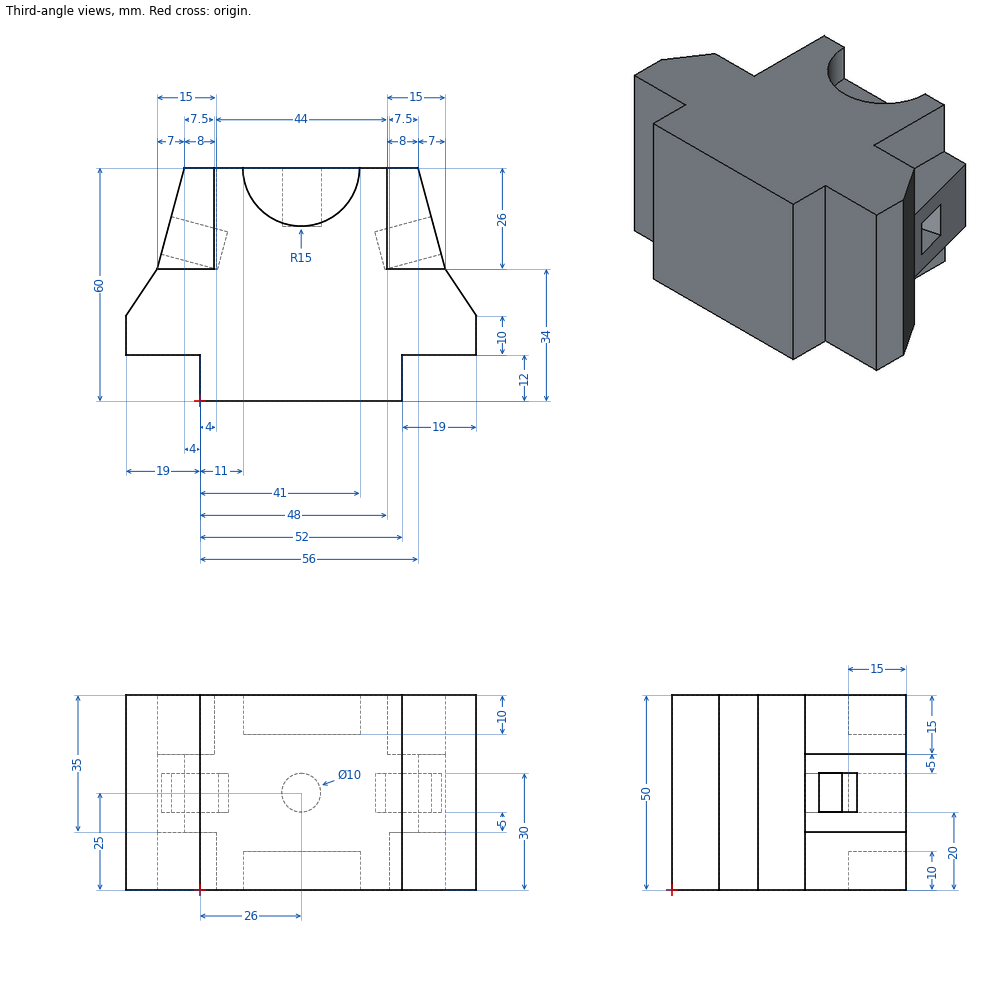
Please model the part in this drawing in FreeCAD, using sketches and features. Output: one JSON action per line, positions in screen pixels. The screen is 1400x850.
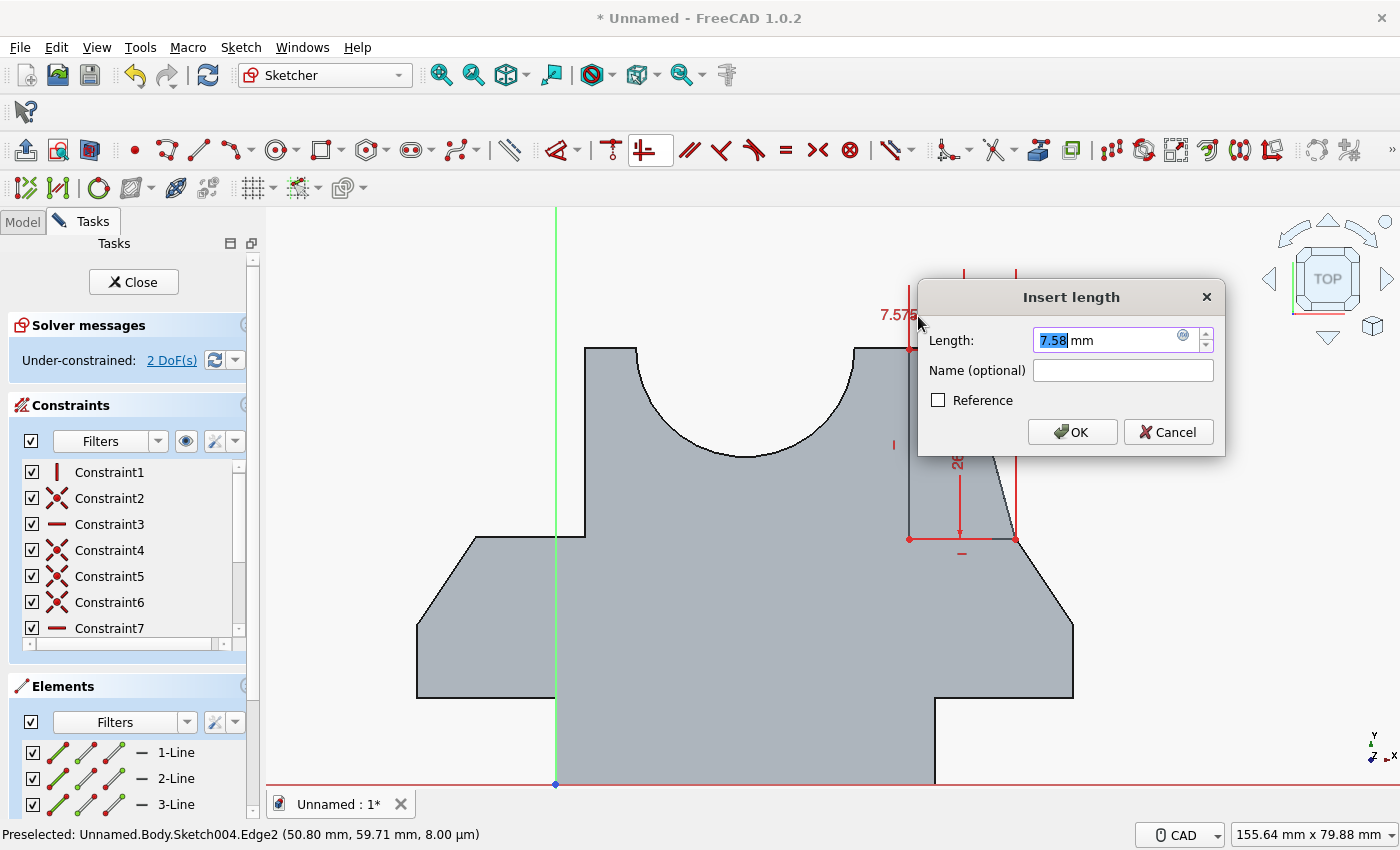
{"action": "type", "text": "7.5"}
{"action": "key", "text": "Return"}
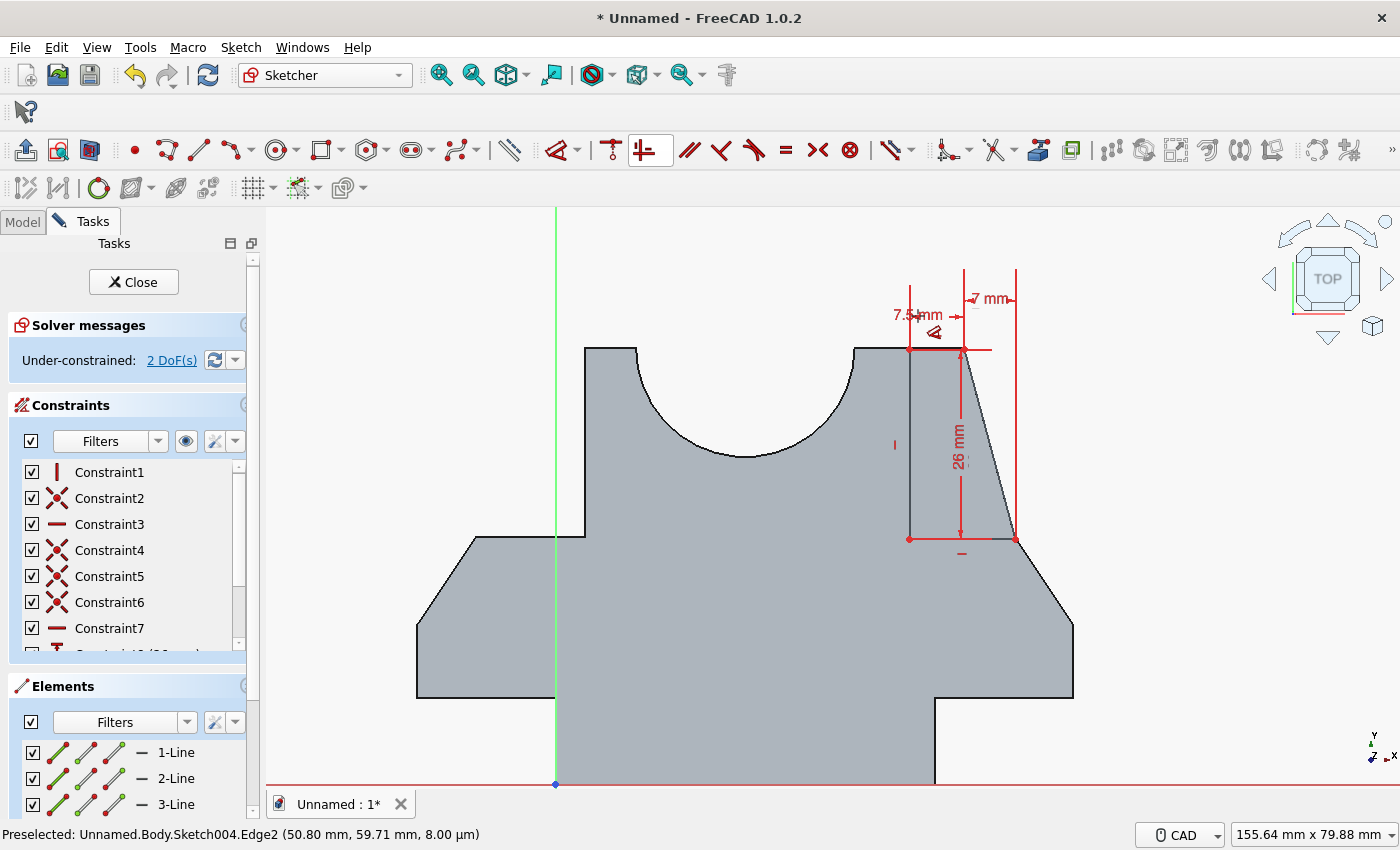
{"action": "left_click", "coordinate": [910, 539]}
{"action": "left_click", "coordinate": [522, 650]}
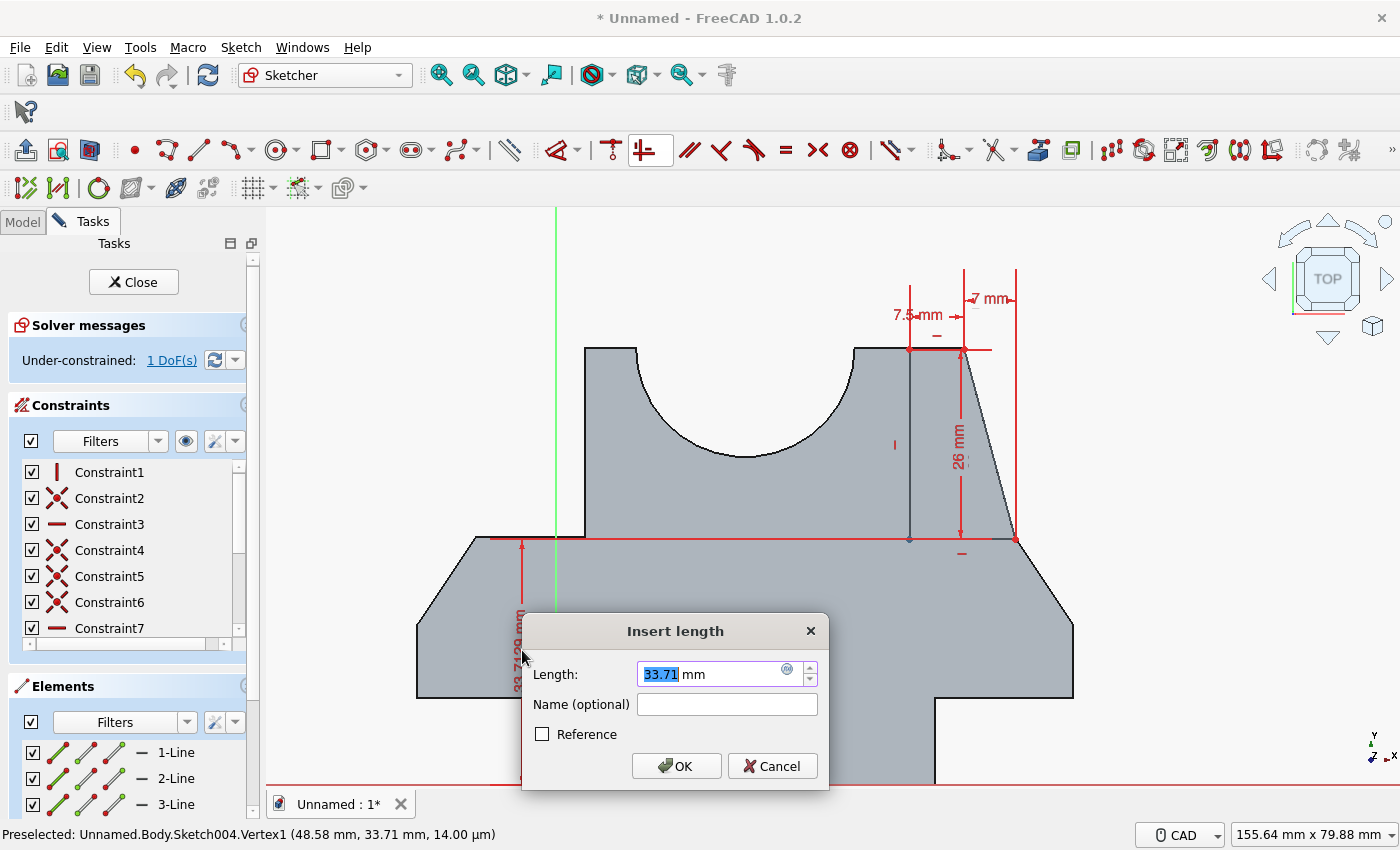
{"action": "type", "text": "34"}
{"action": "key", "text": "Return"}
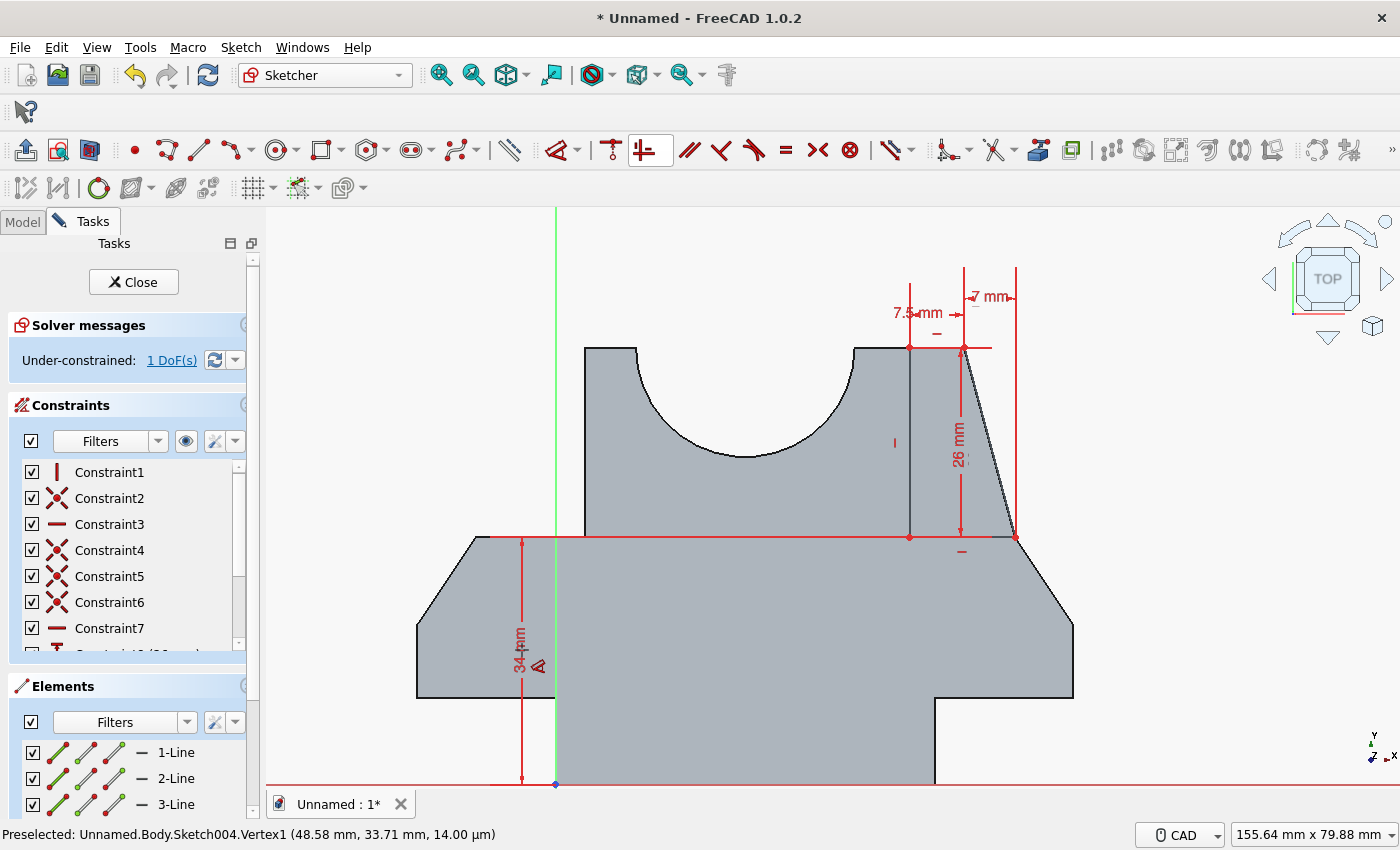
{"action": "left_click", "coordinate": [965, 348]}
{"action": "left_click", "coordinate": [760, 314]}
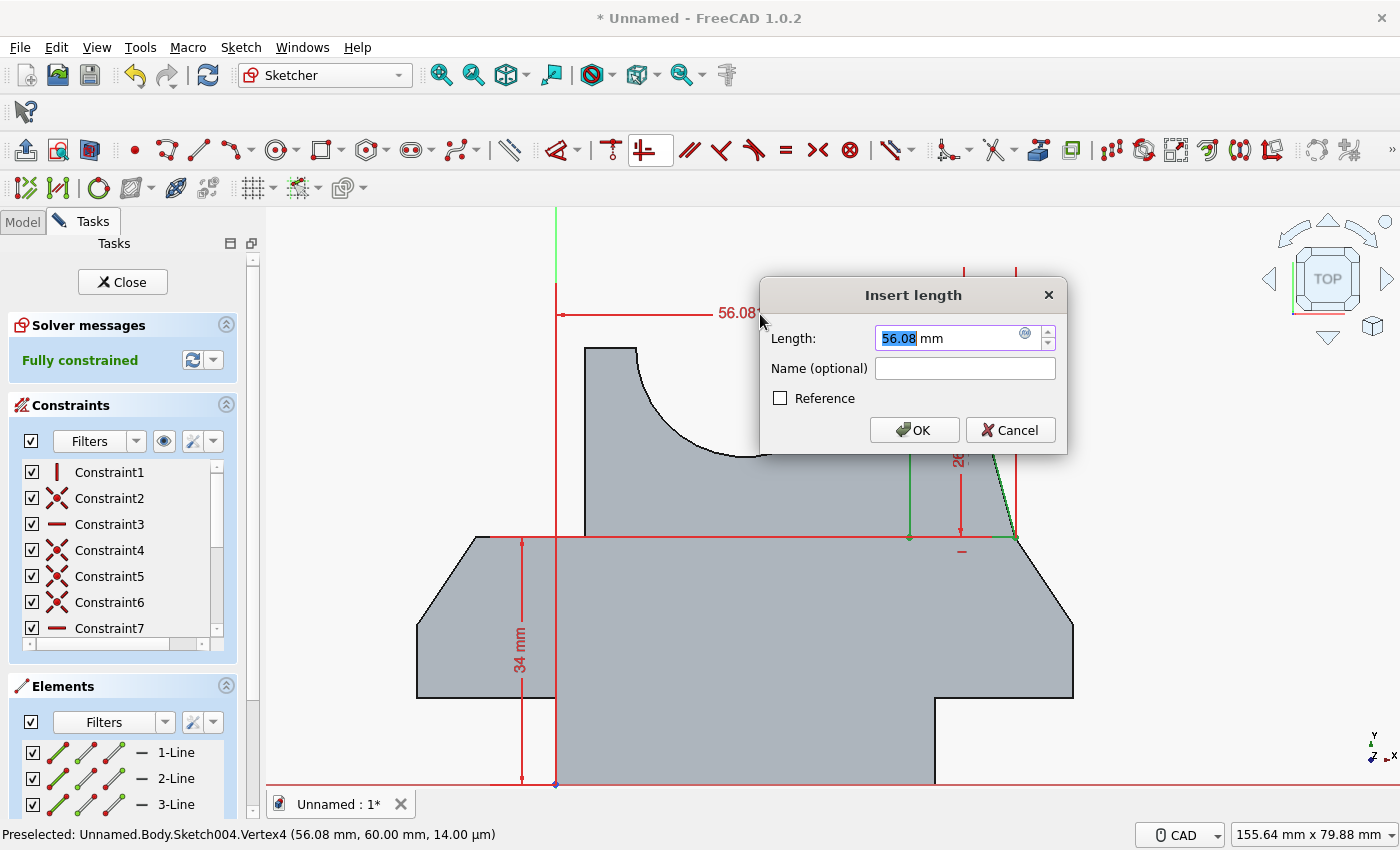
{"action": "type", "text": "56"}
{"action": "key", "text": "Return"}
{"action": "key", "text": "Escape"}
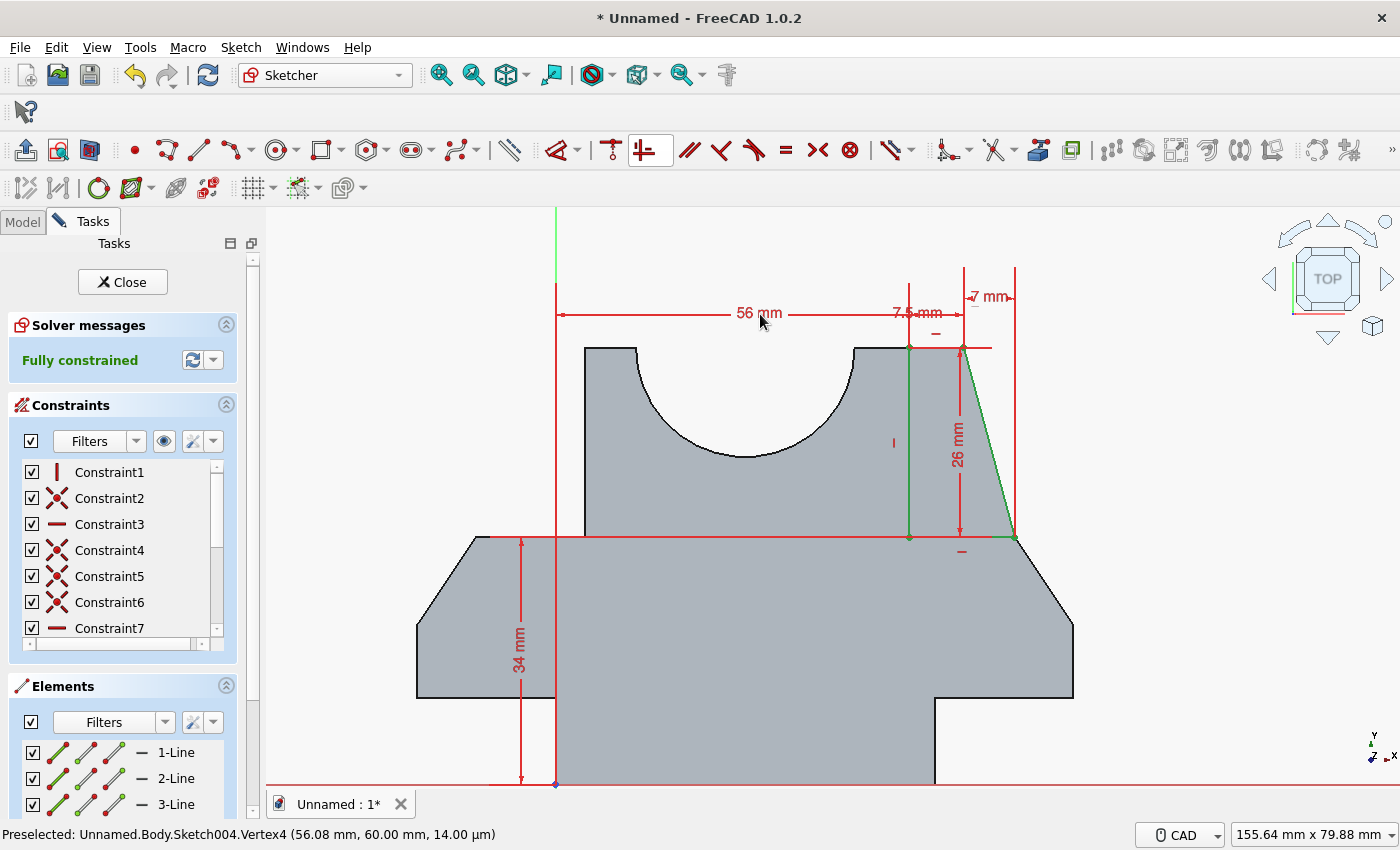
{"action": "left_click", "coordinate": [123, 282]}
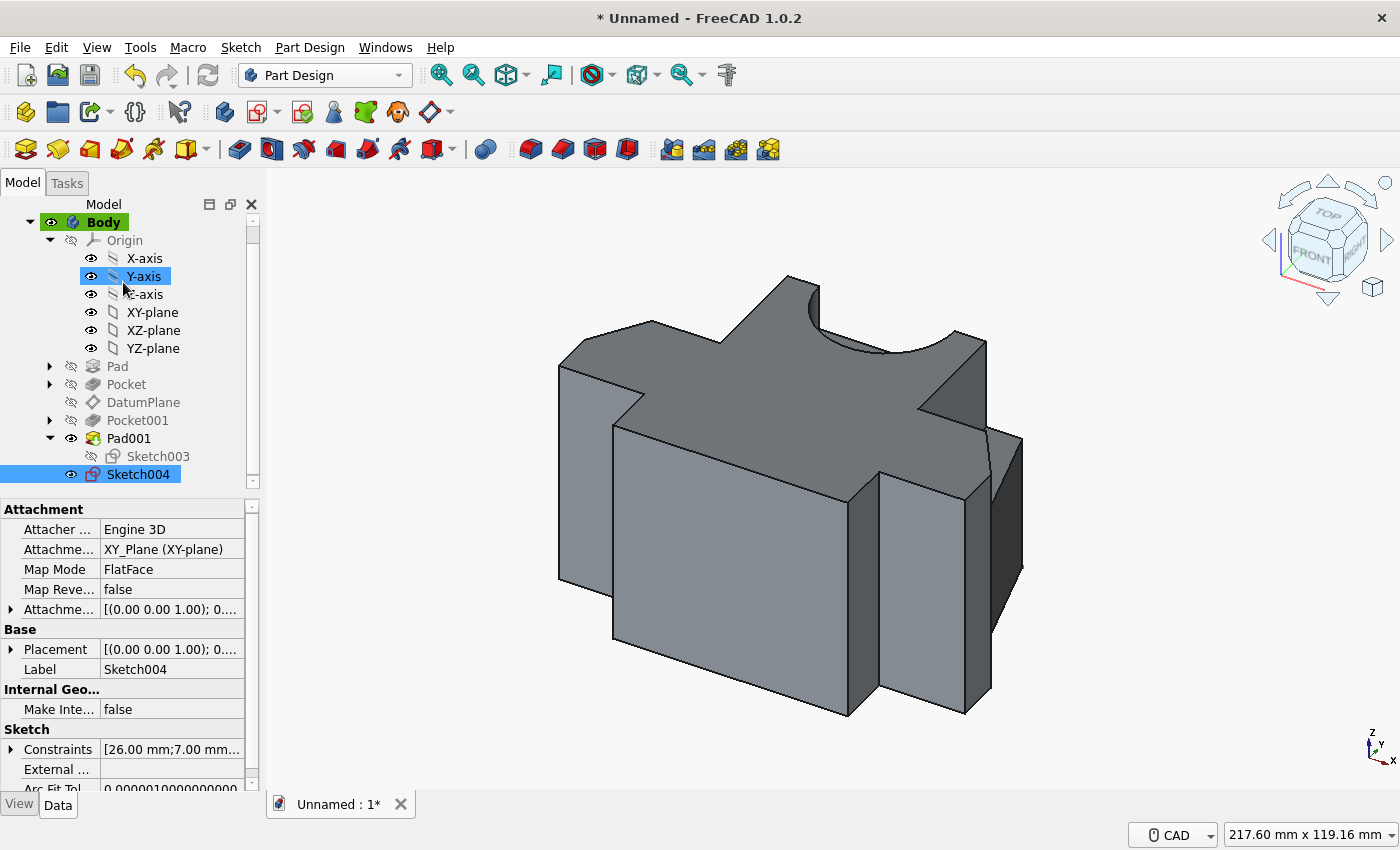
{"action": "left_click", "coordinate": [240, 150]}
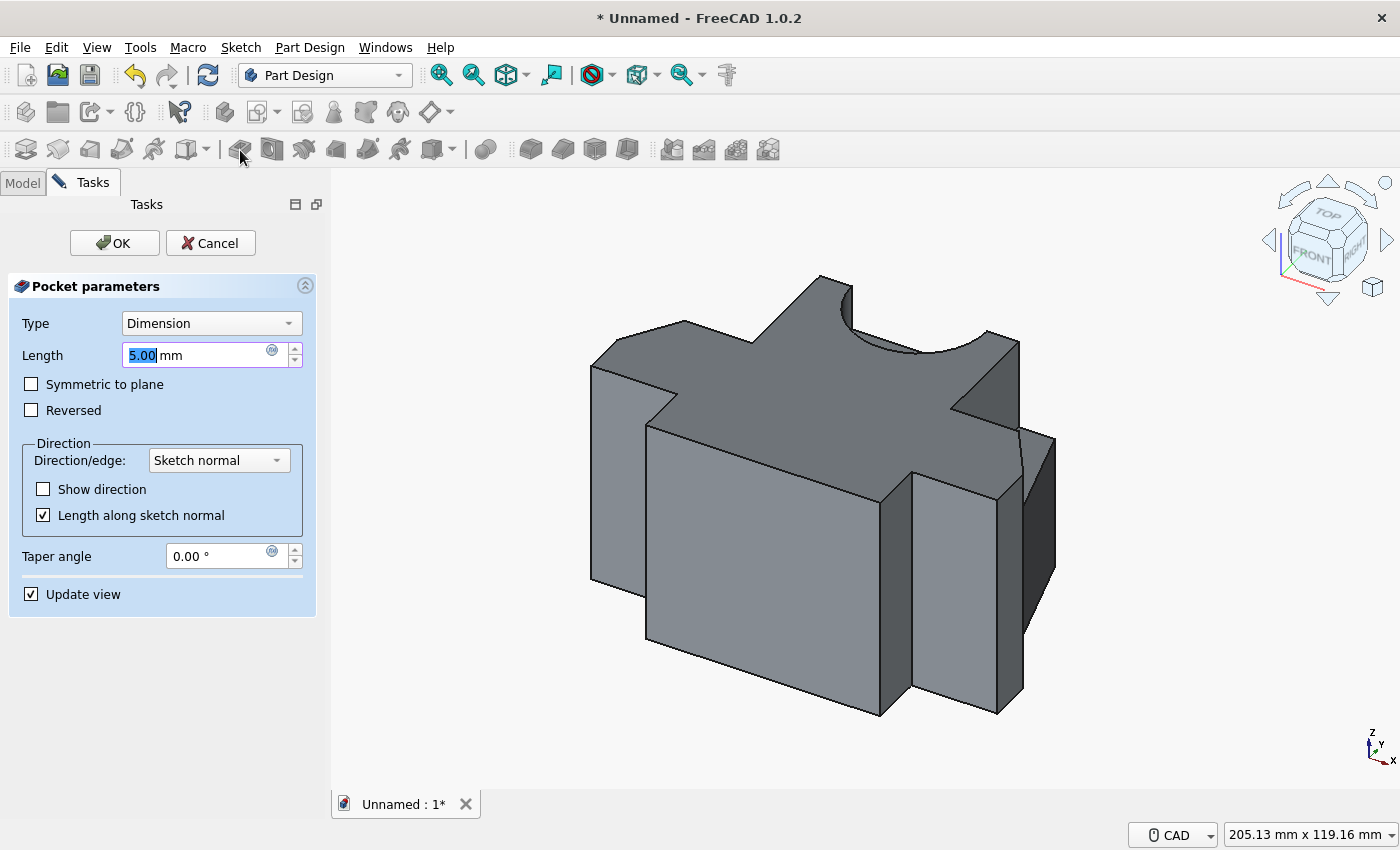
{"action": "type", "text": "20"}
{"action": "key", "text": "Tab"}